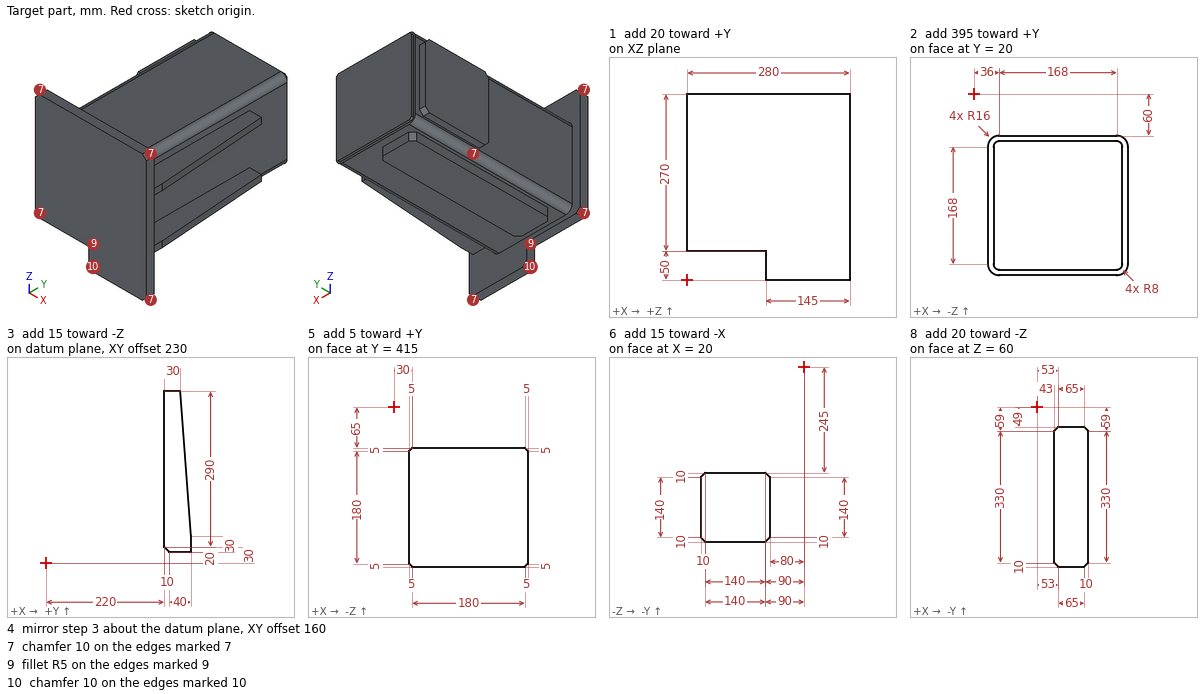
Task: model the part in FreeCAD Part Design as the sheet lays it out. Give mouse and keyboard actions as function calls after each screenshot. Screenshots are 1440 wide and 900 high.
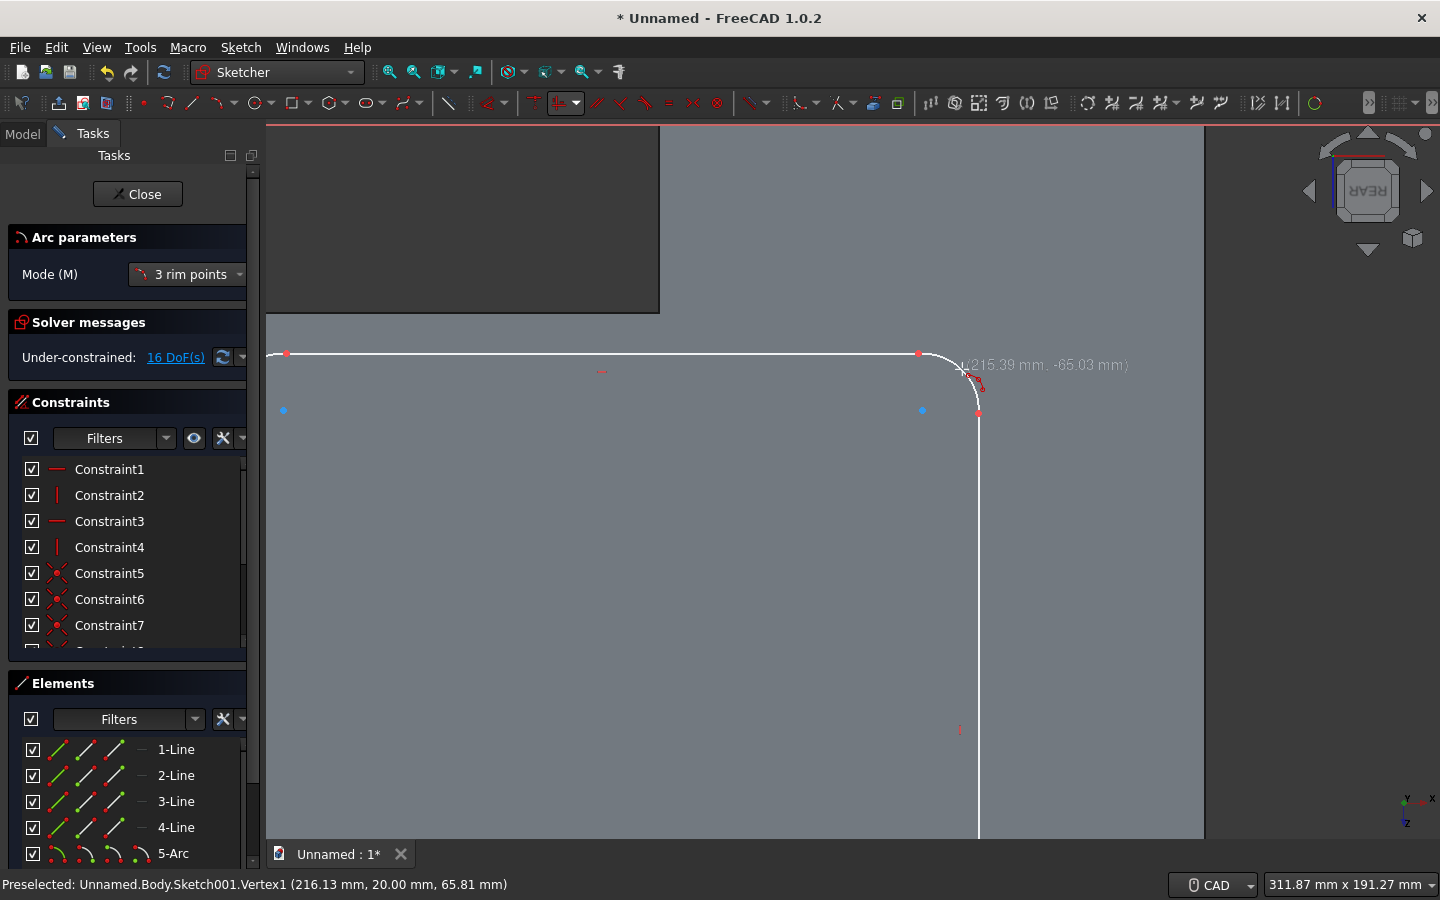
click(192, 104)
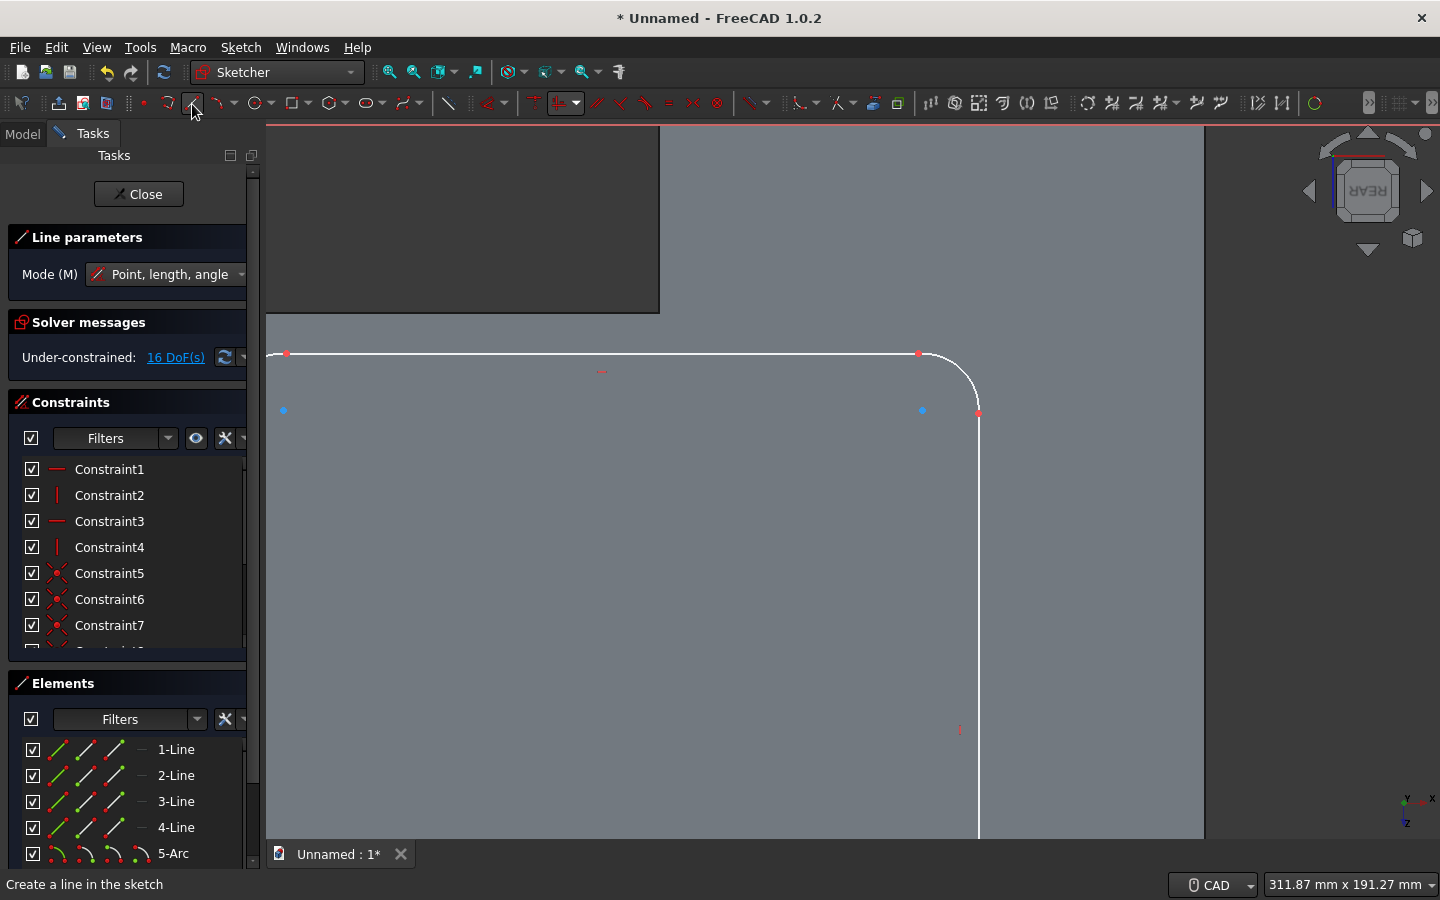
scroll(963, 368, down, 4)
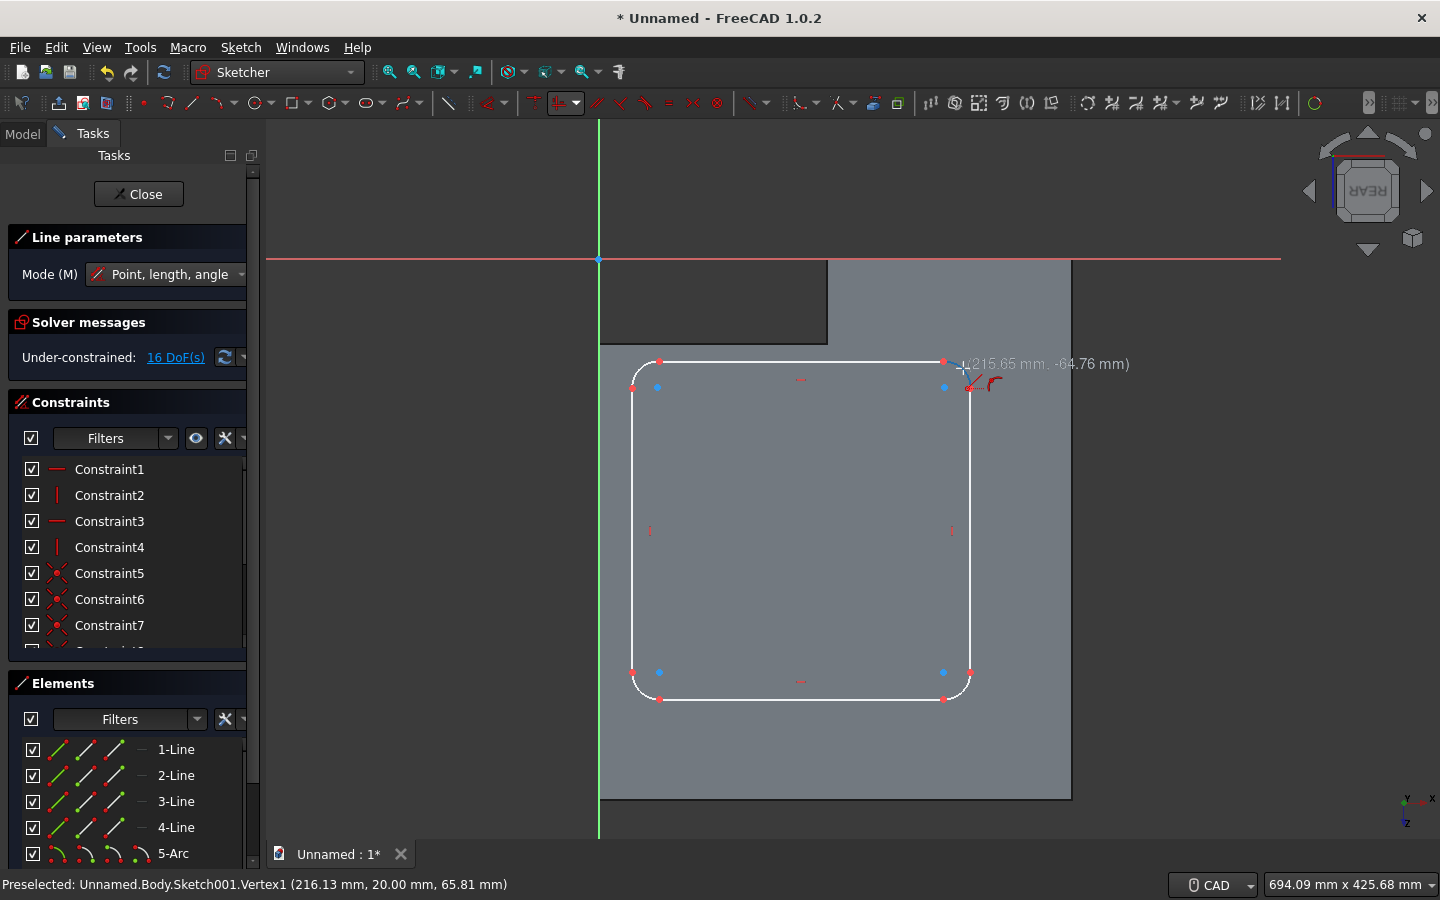
click(659, 374)
click(944, 374)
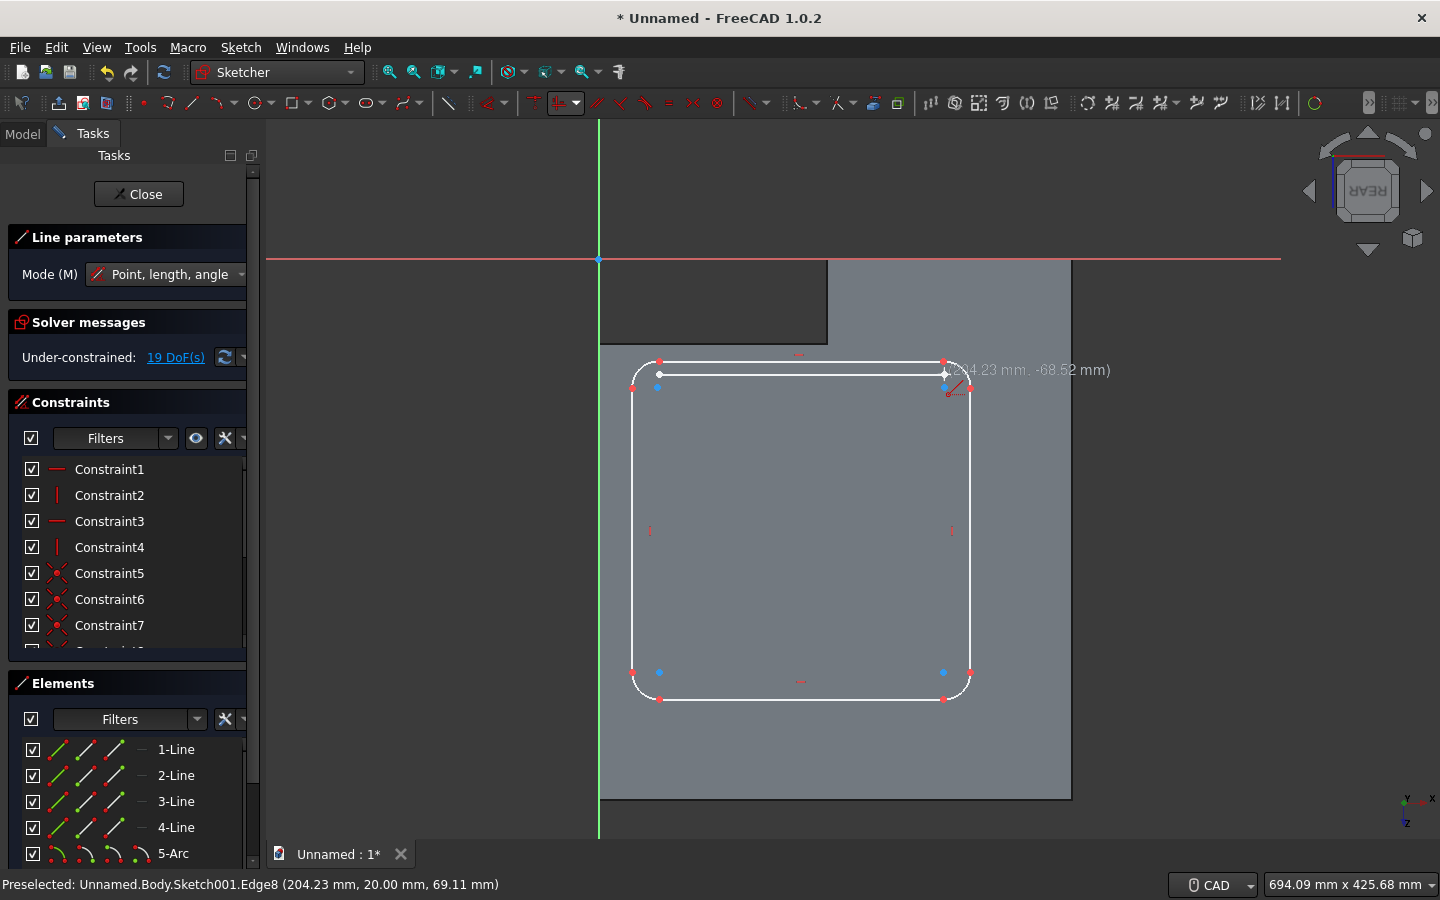
click(957, 388)
click(957, 672)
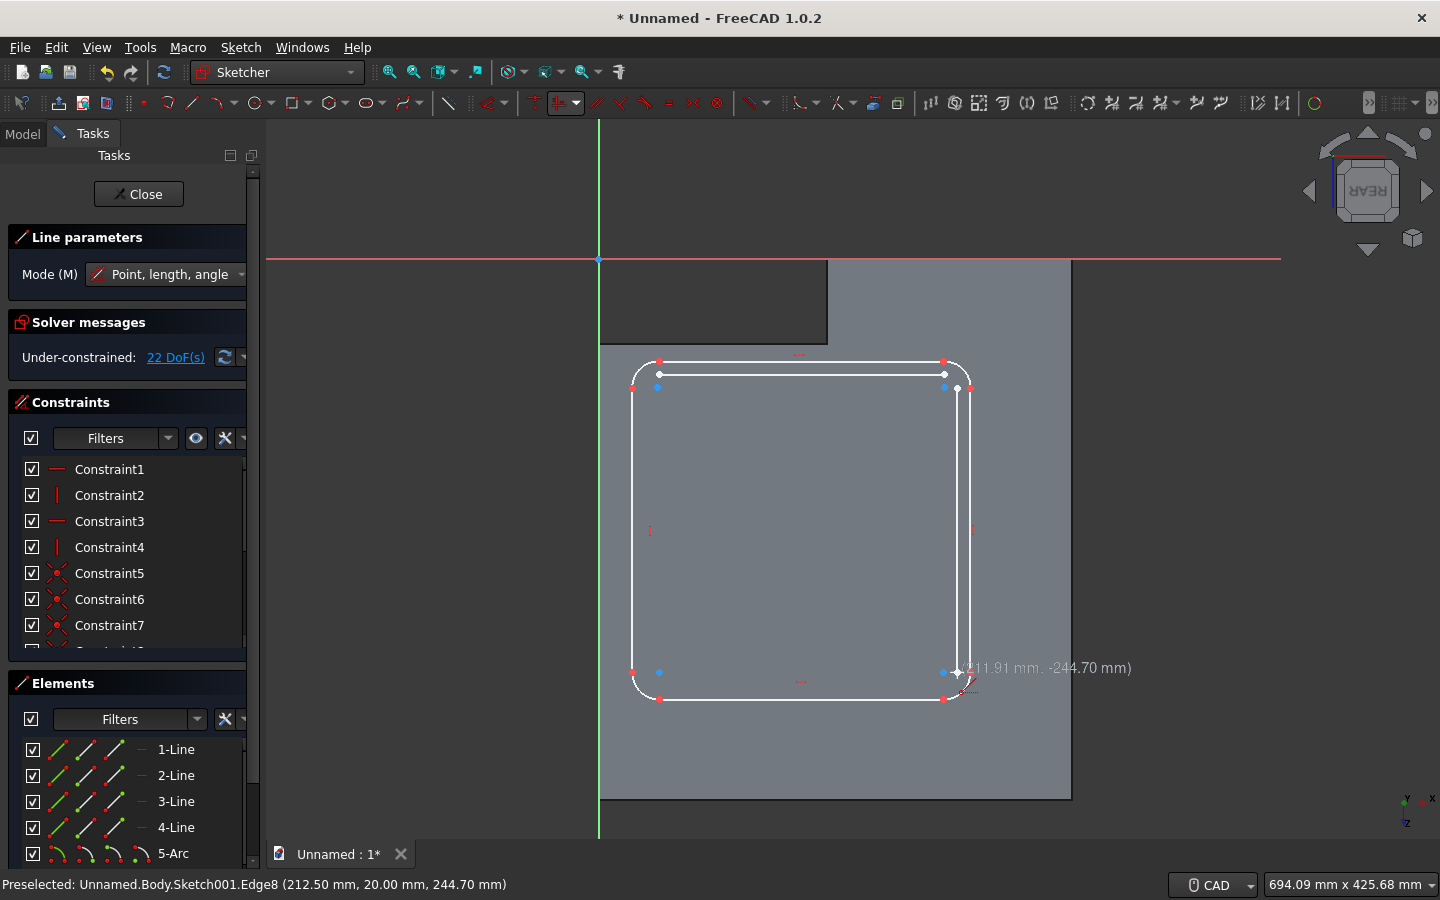
click(944, 685)
click(659, 685)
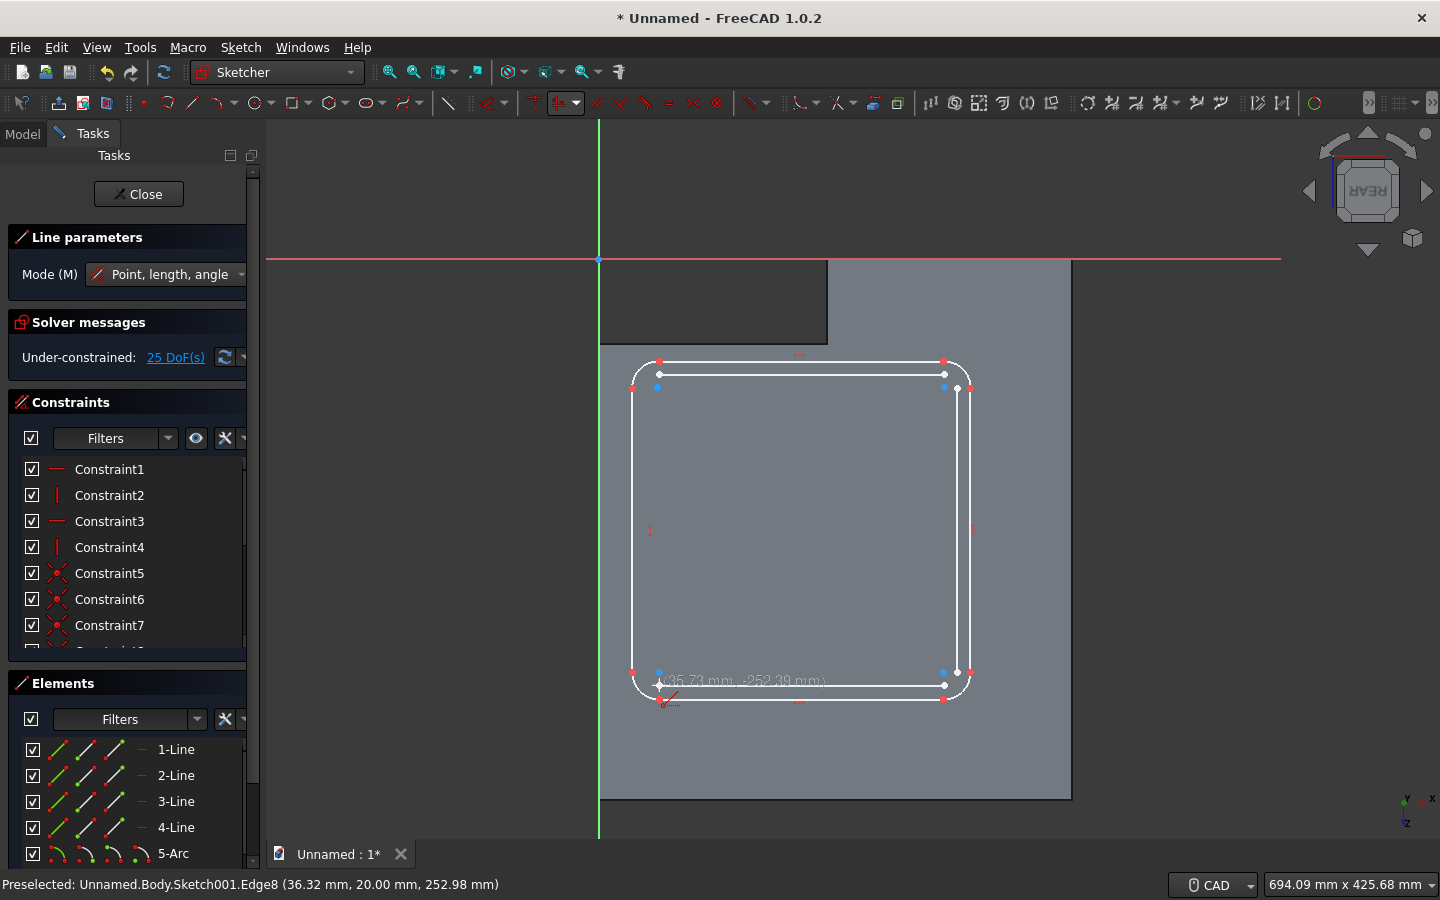
click(646, 672)
click(646, 388)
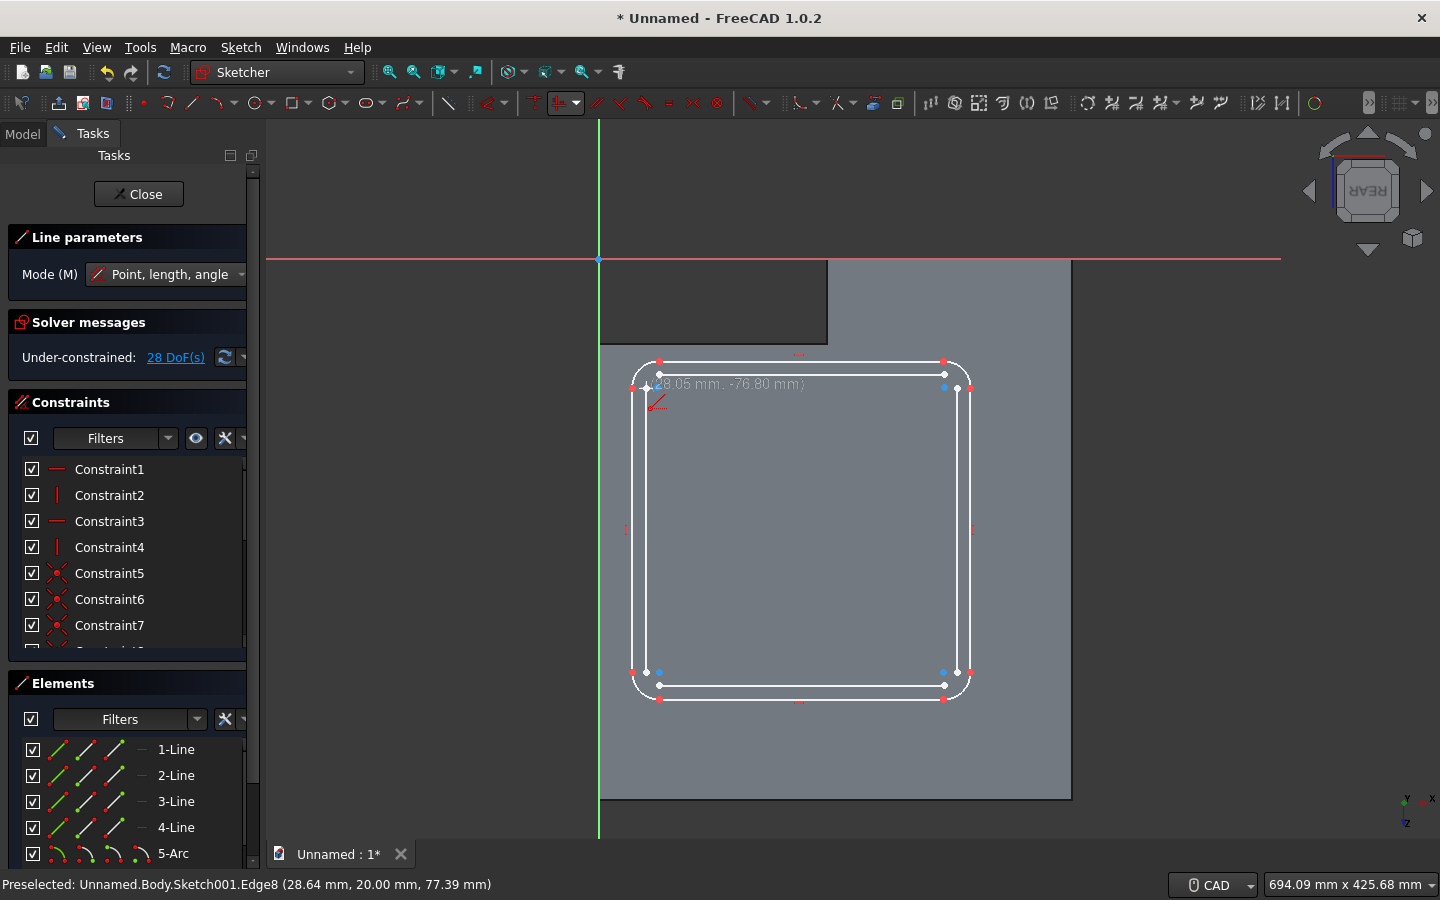
click(218, 104)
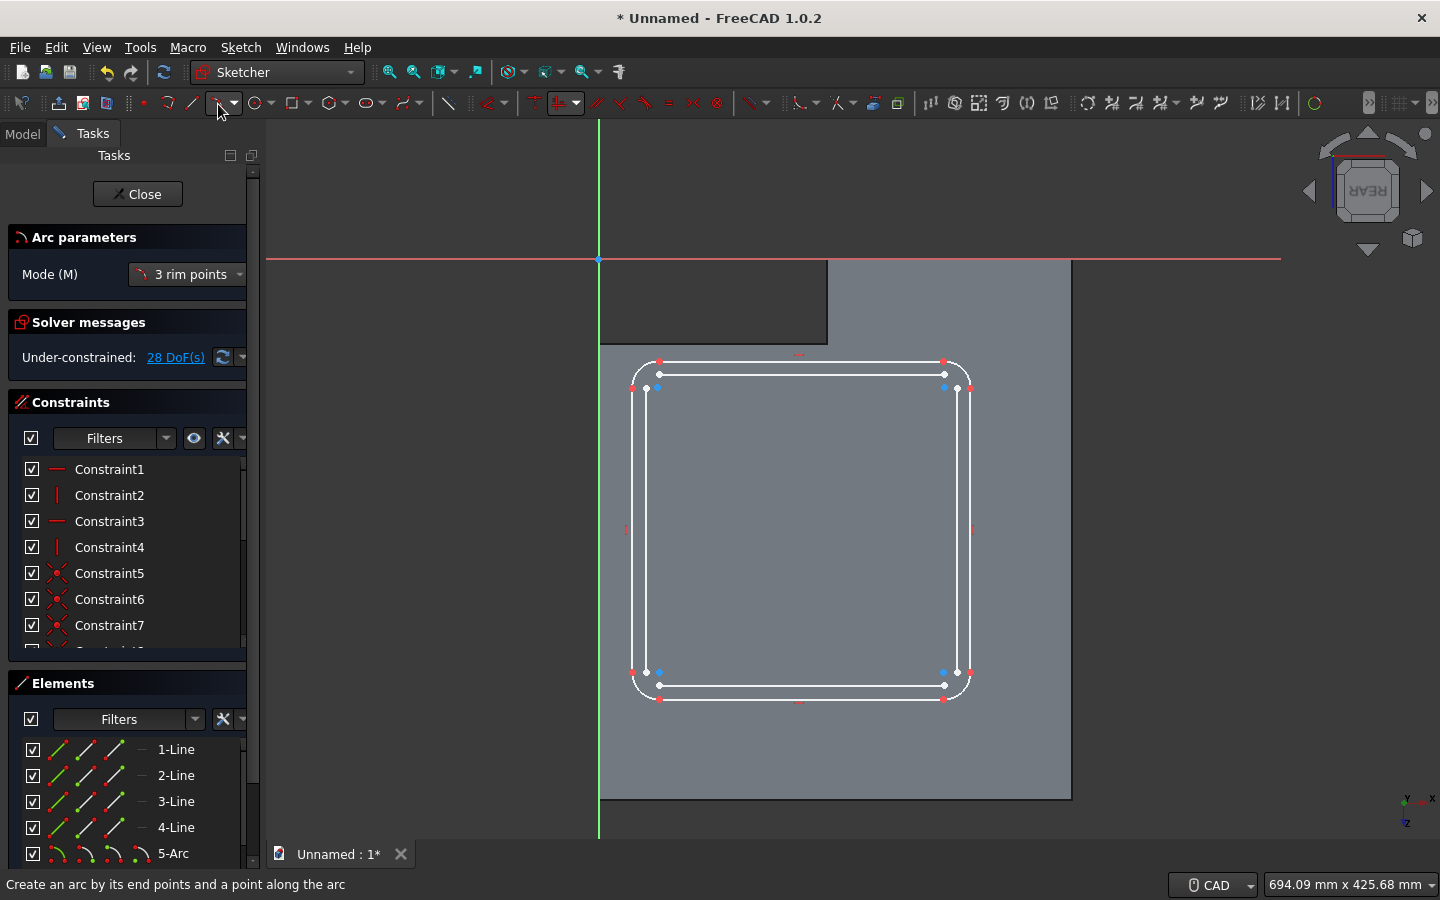
click(944, 375)
click(957, 389)